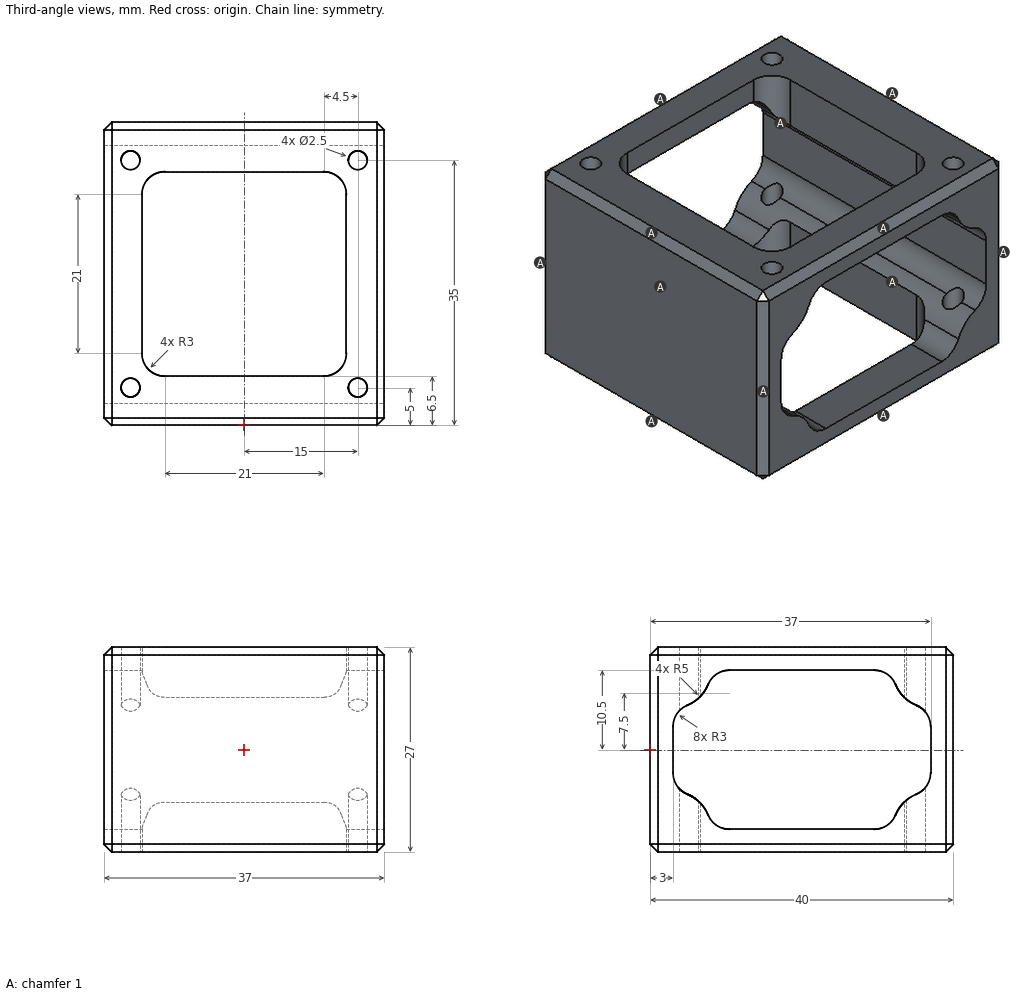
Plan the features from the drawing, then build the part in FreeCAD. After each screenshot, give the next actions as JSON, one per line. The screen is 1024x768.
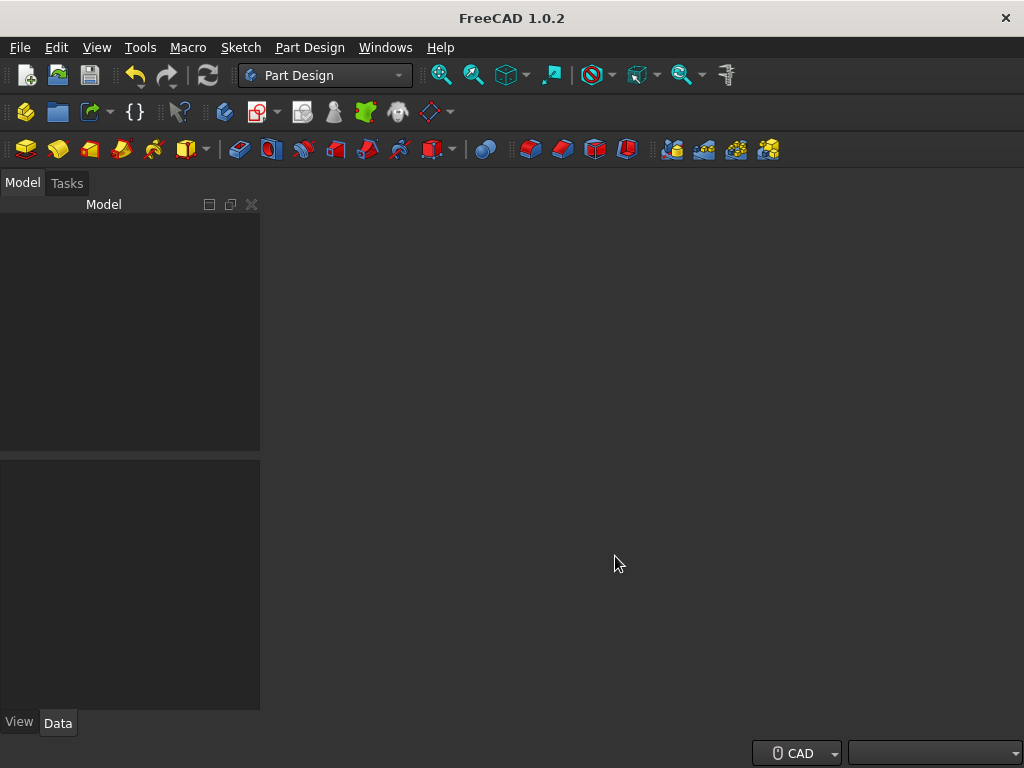
{"action": "key", "text": "ctrl+n"}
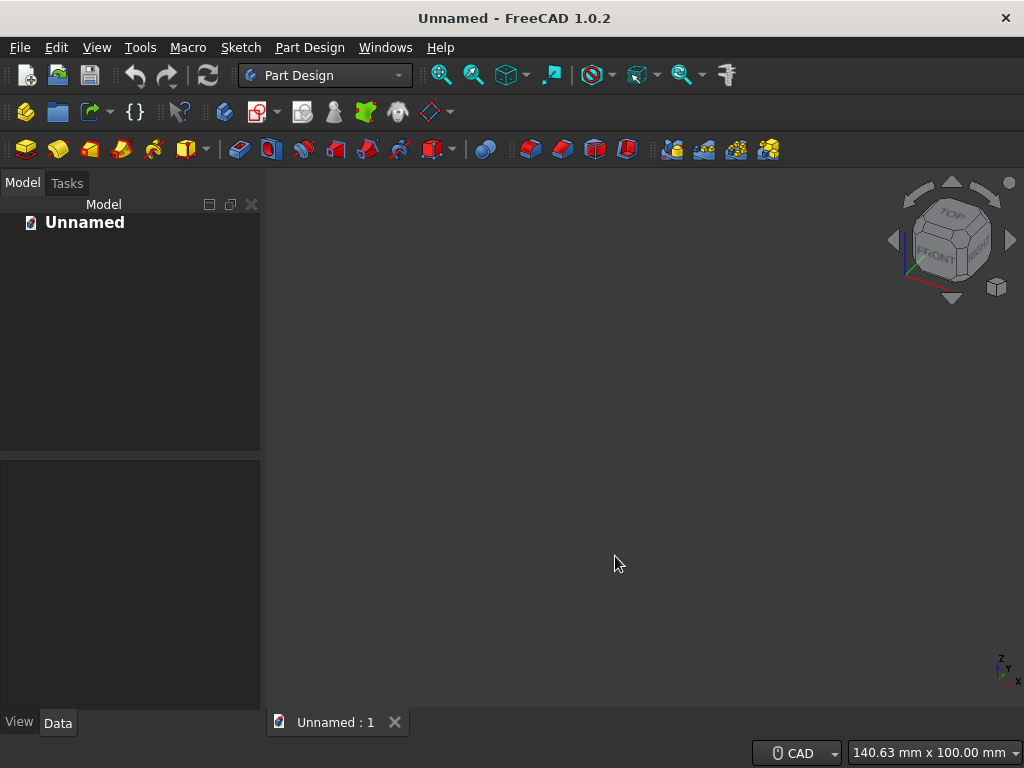
{"action": "left_click", "coordinate": [258, 112]}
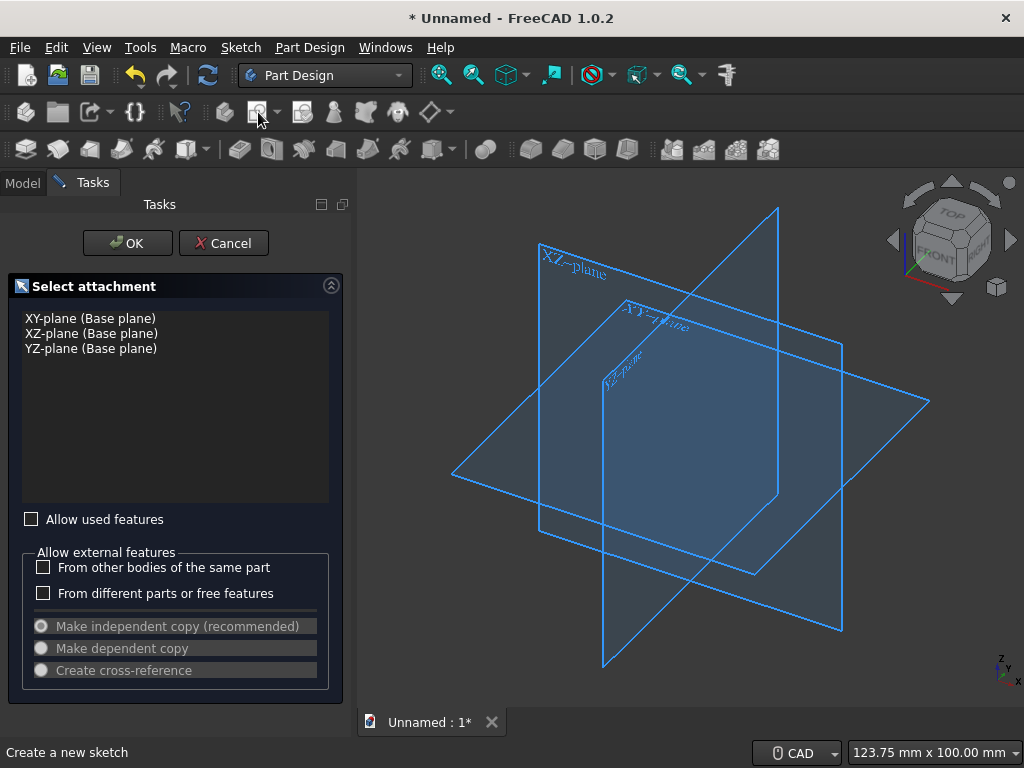
{"action": "left_click", "coordinate": [82, 334]}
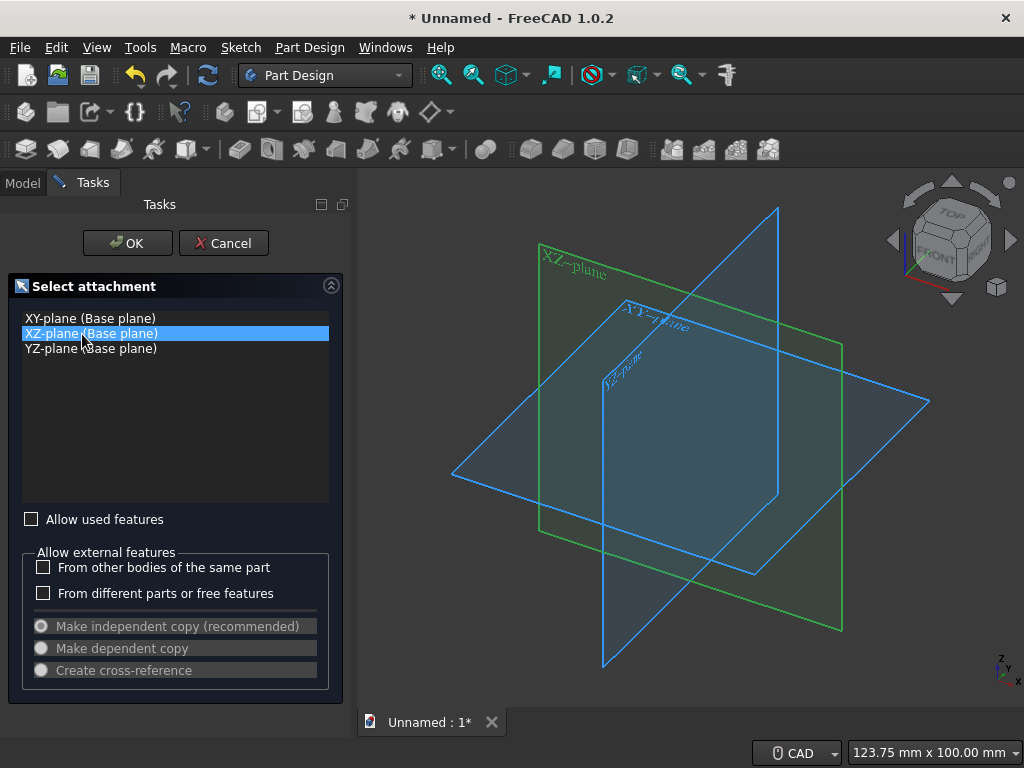
{"action": "left_click", "coordinate": [128, 243]}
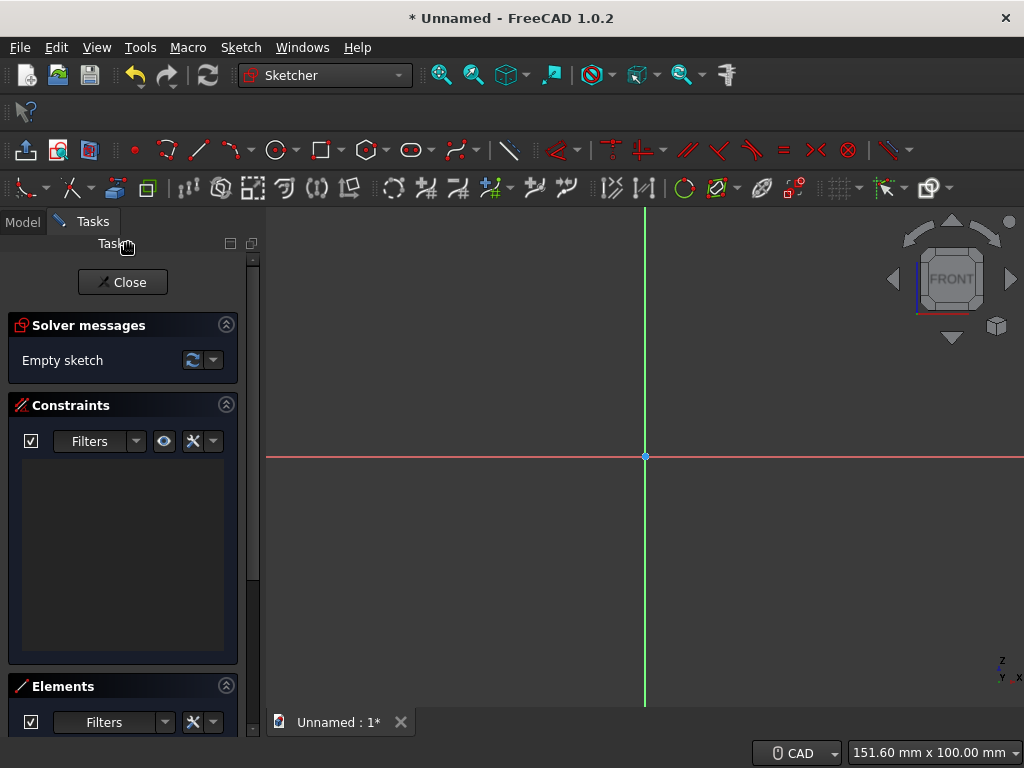
{"action": "scroll", "coordinate": [701, 457], "scroll_direction": "up", "scroll_amount": 4}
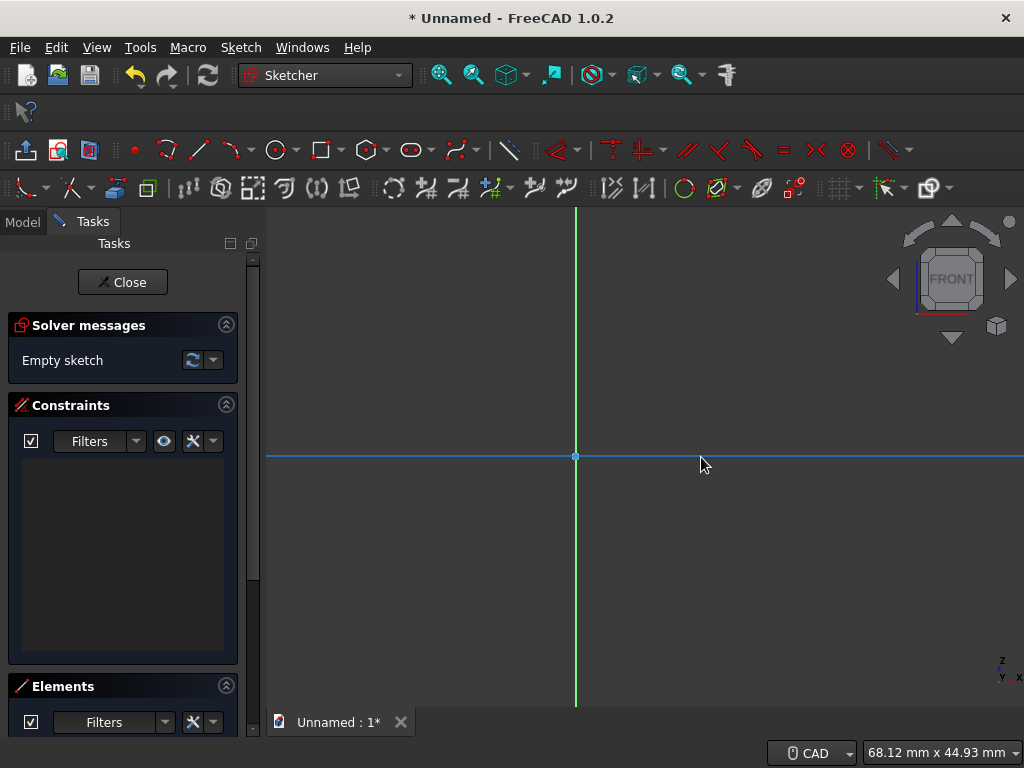
{"action": "key", "text": "g v"}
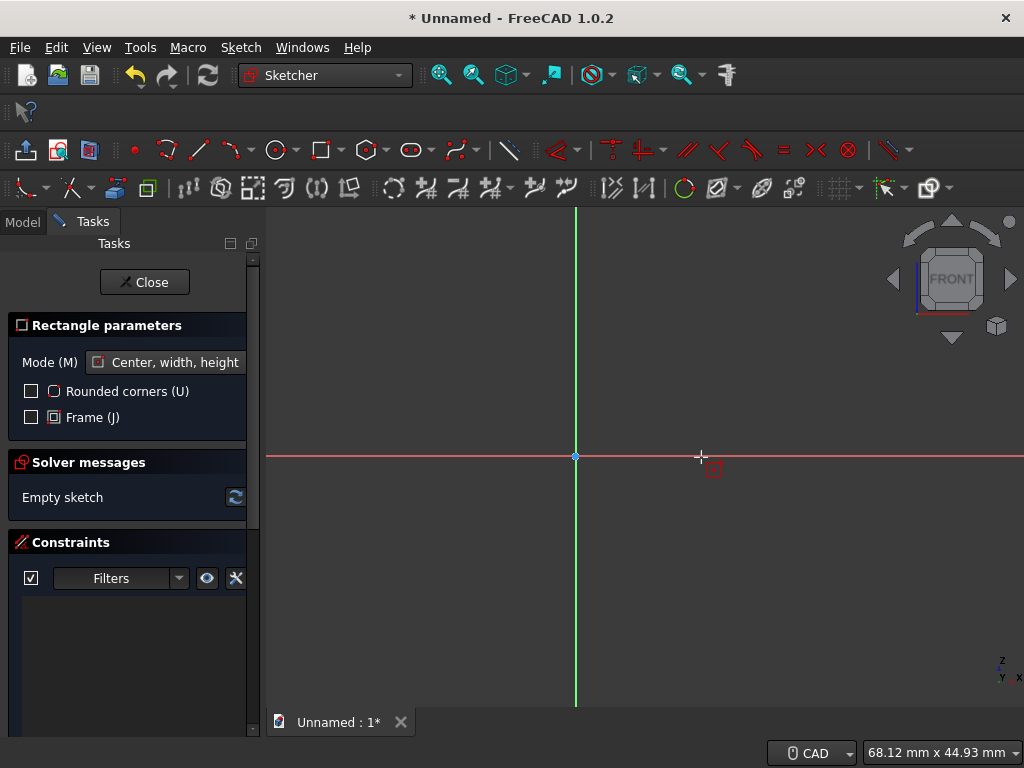
{"action": "left_click", "coordinate": [576, 456]}
{"action": "left_click", "coordinate": [782, 306]}
{"action": "key", "text": "Escape"}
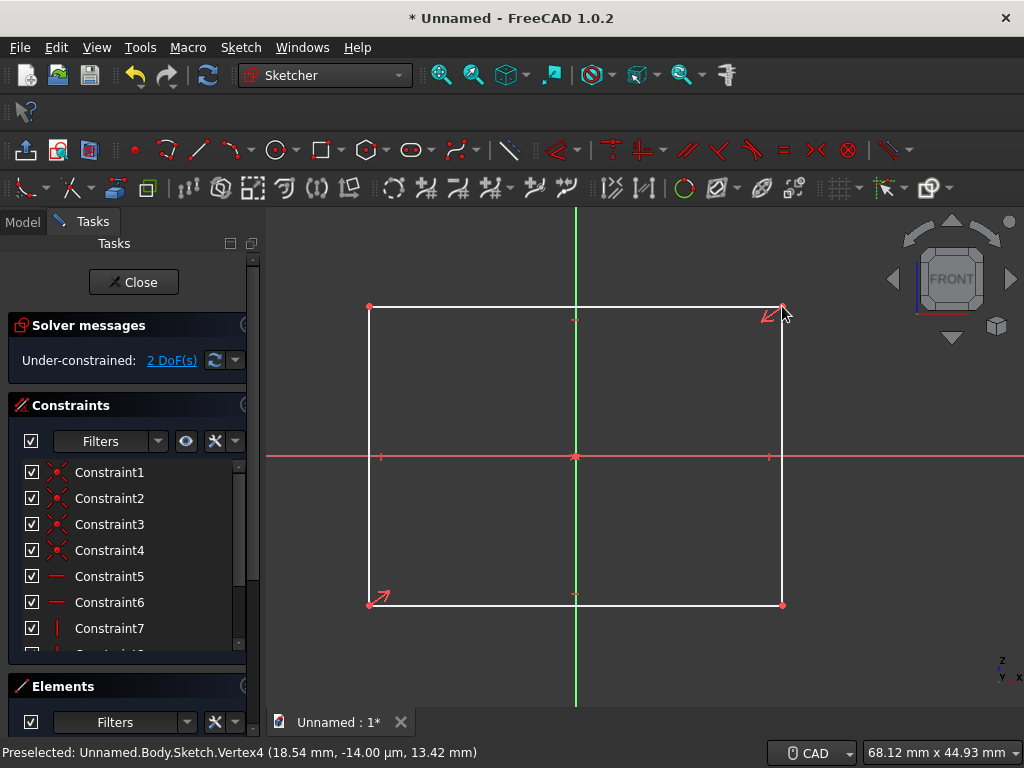
{"action": "key", "text": "d"}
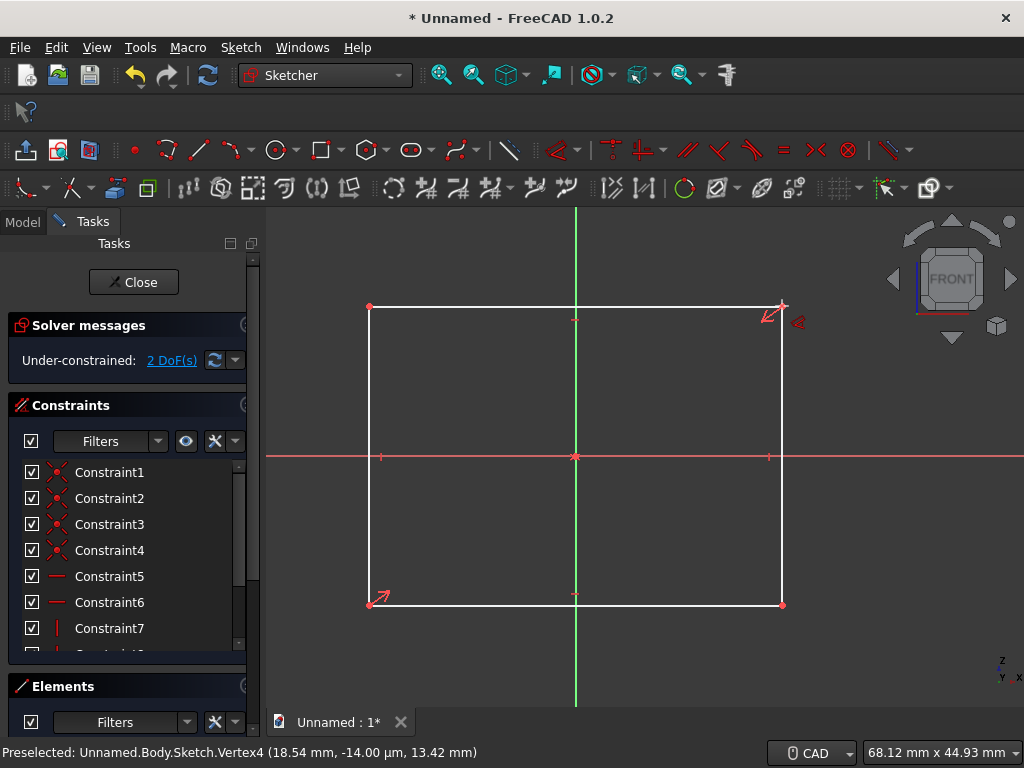
{"action": "left_click", "coordinate": [493, 606]}
{"action": "left_click", "coordinate": [481, 640]}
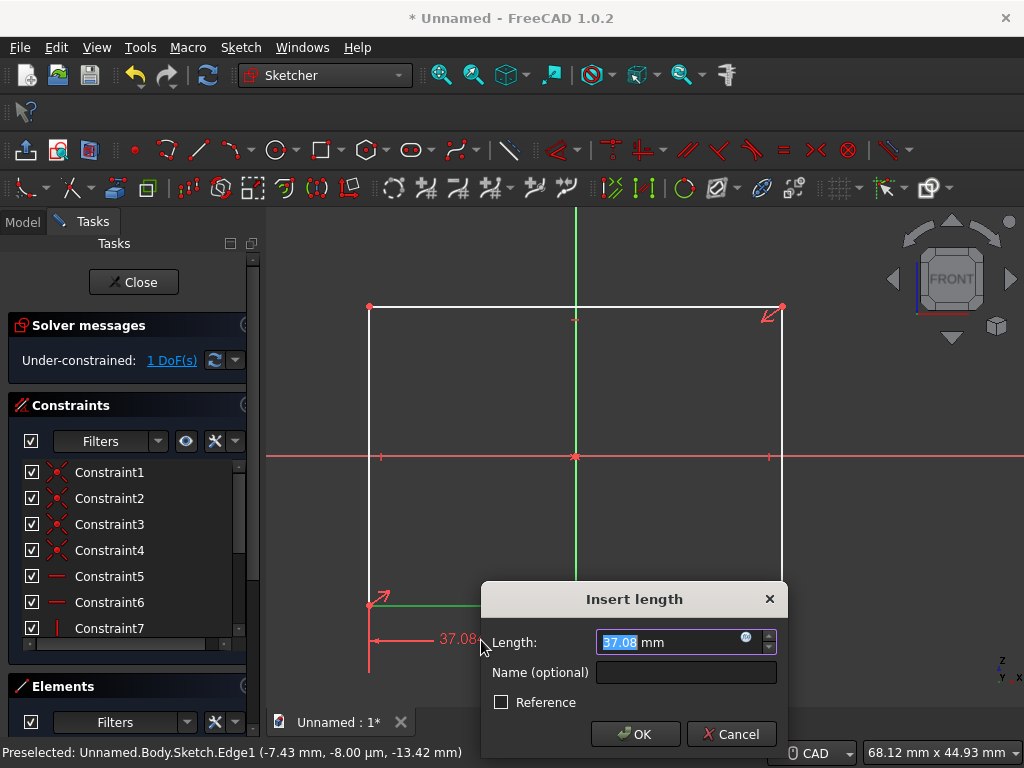
{"action": "type", "text": "37"}
{"action": "key", "text": "Return"}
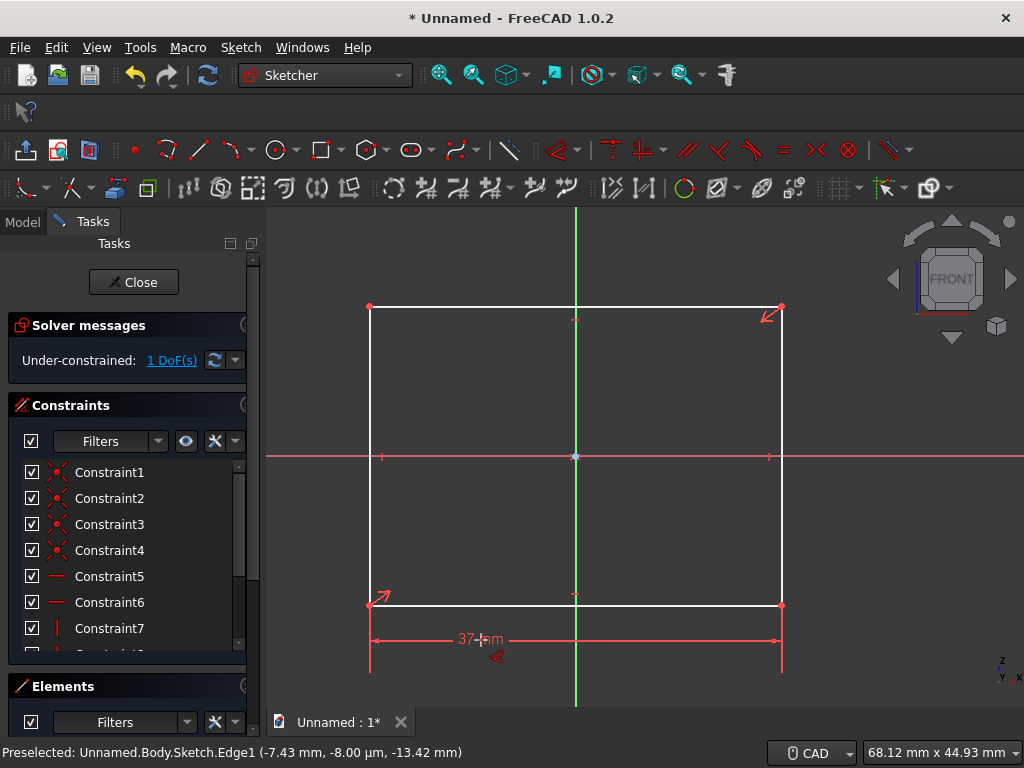
{"action": "left_click", "coordinate": [782, 516]}
{"action": "left_click", "coordinate": [816, 388]}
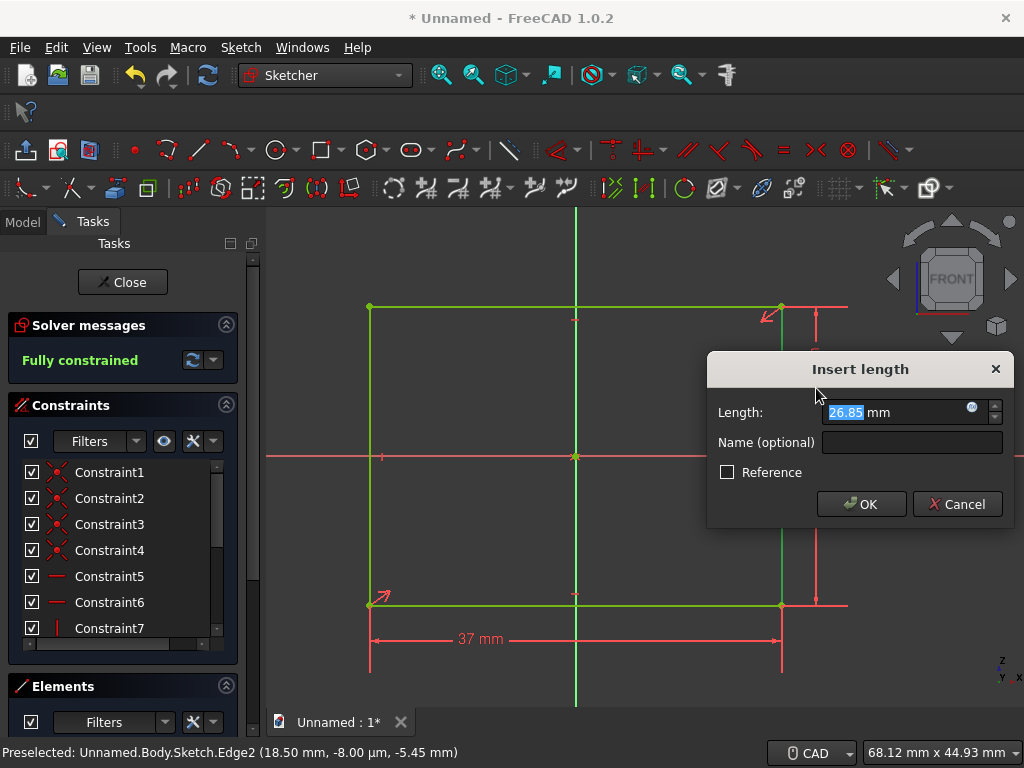
{"action": "type", "text": "27"}
{"action": "key", "text": "Return"}
{"action": "key", "text": "Escape"}